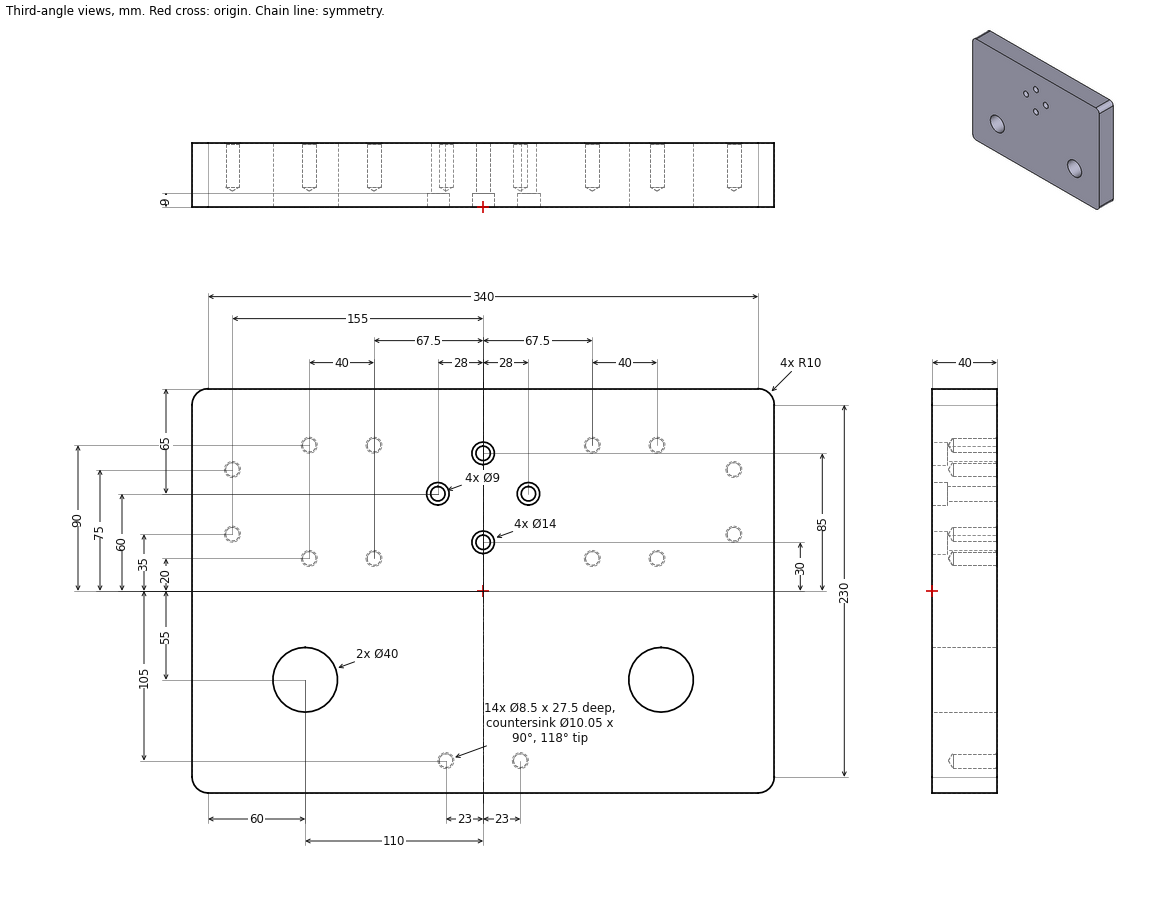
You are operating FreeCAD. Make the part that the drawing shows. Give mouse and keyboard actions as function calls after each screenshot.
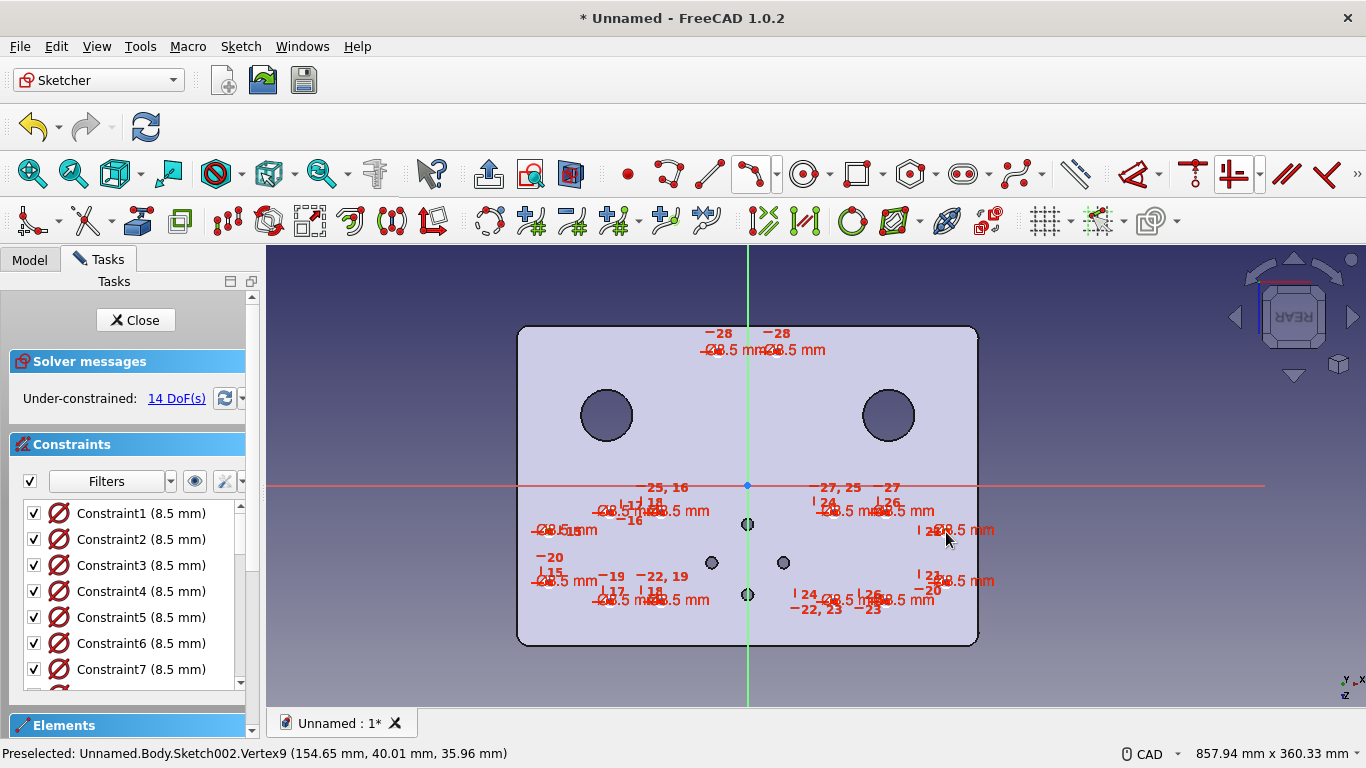
click(748, 650)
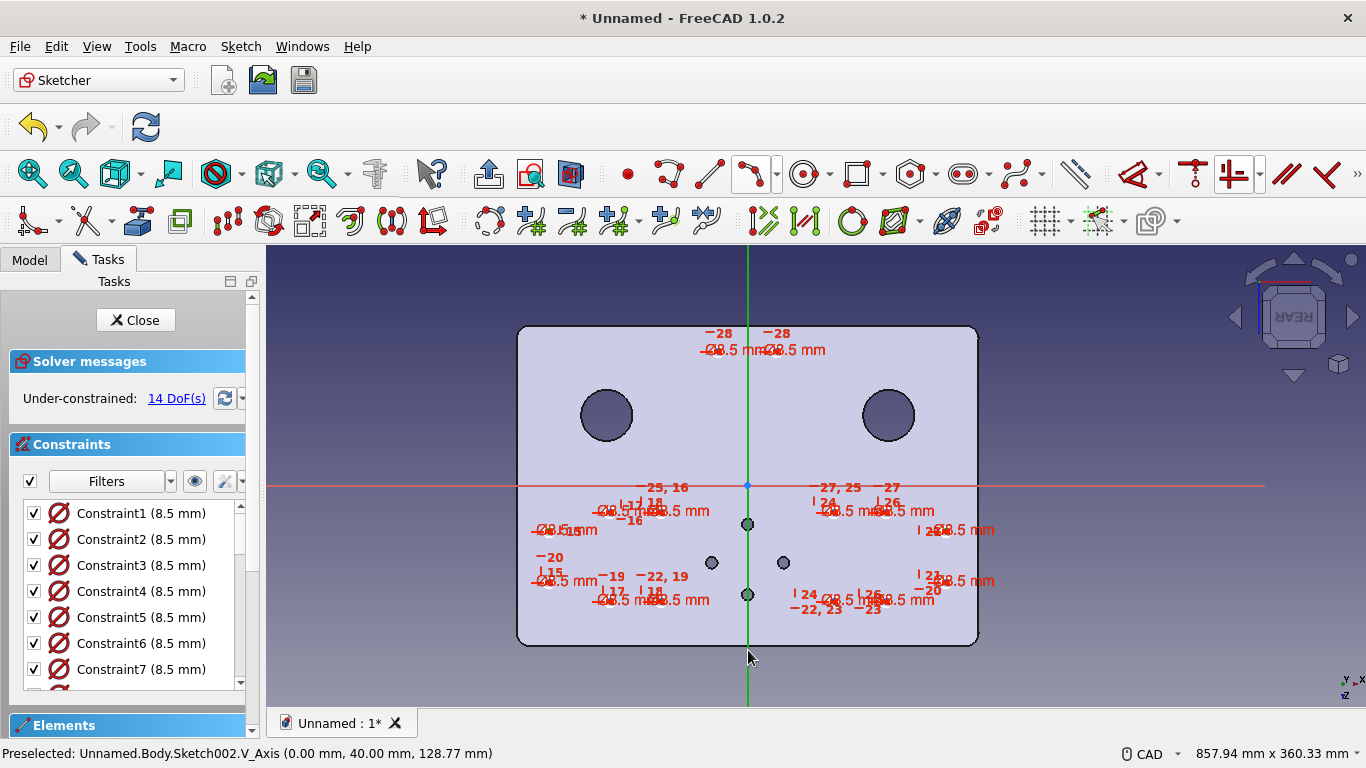
key(s)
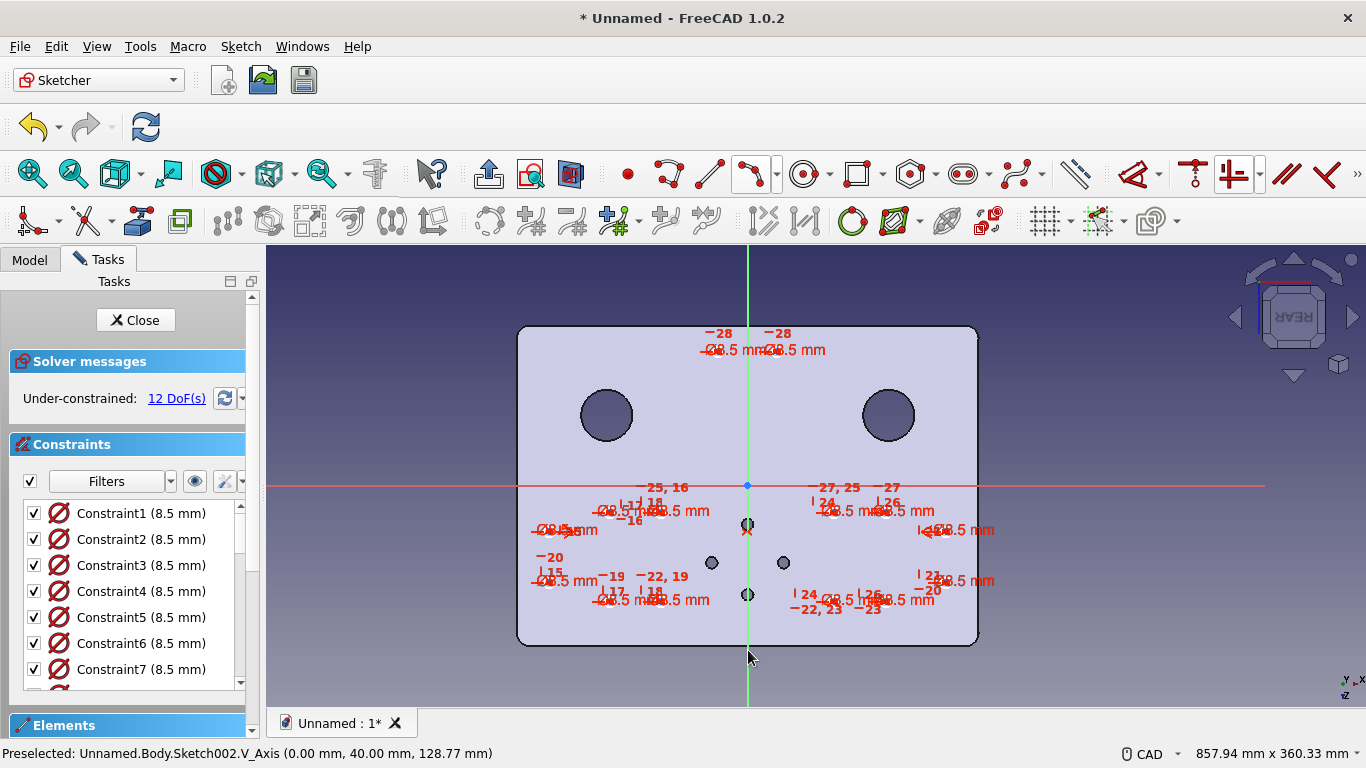
click(1132, 174)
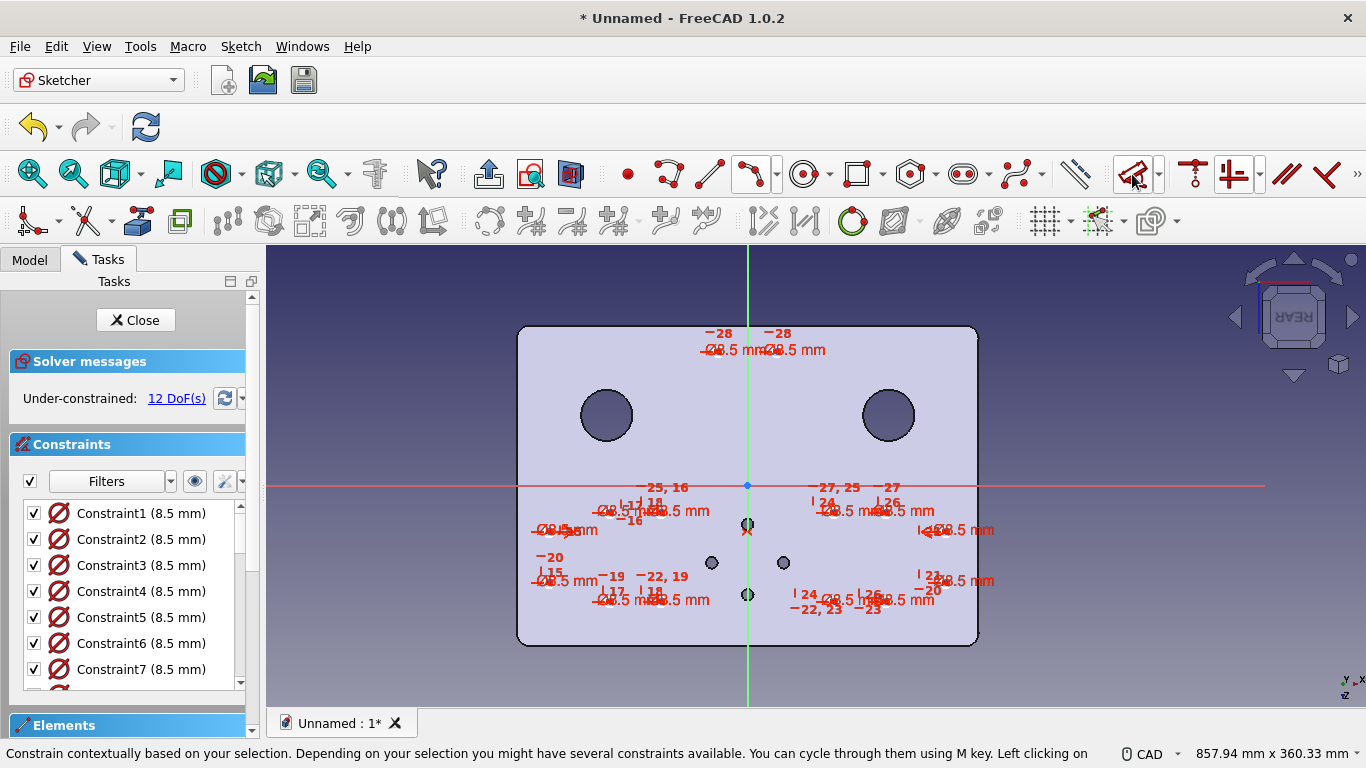
scroll(718, 352, up, 2)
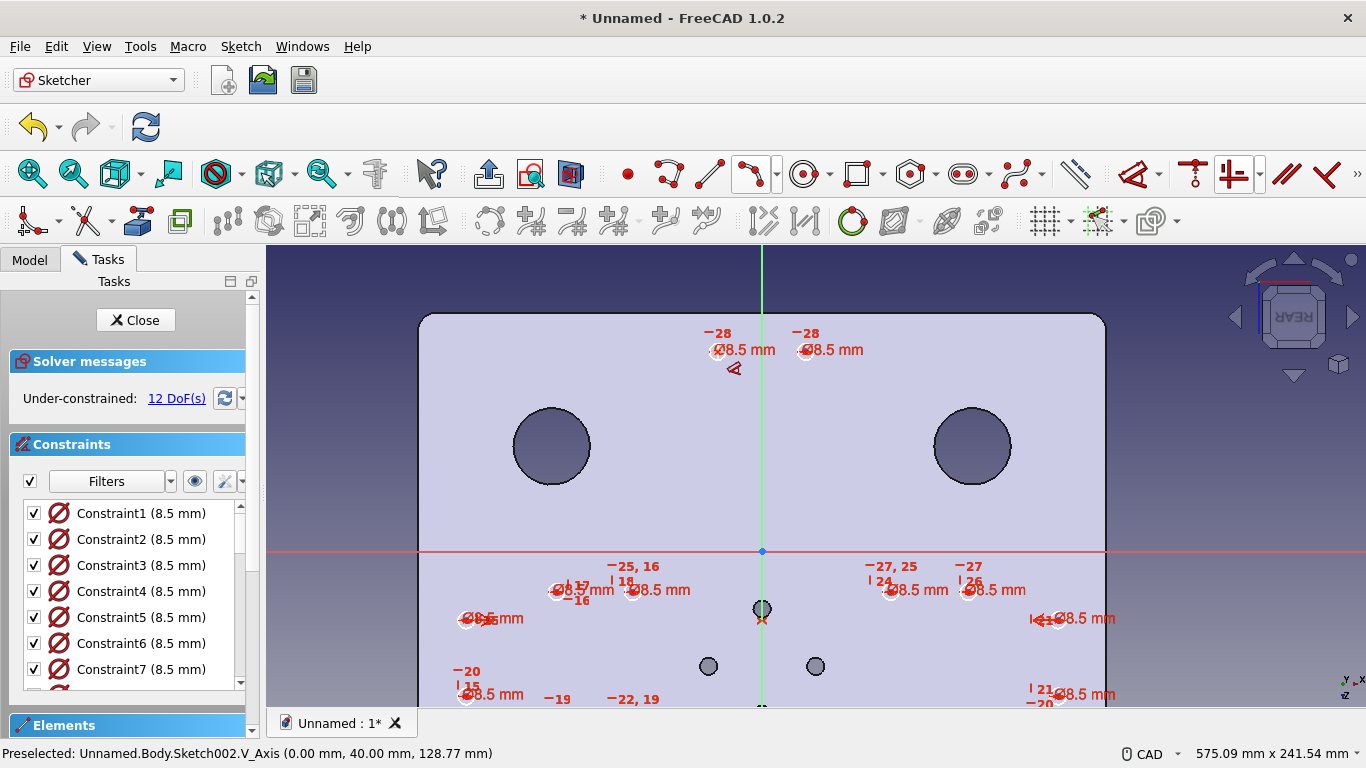
click(718, 352)
click(740, 318)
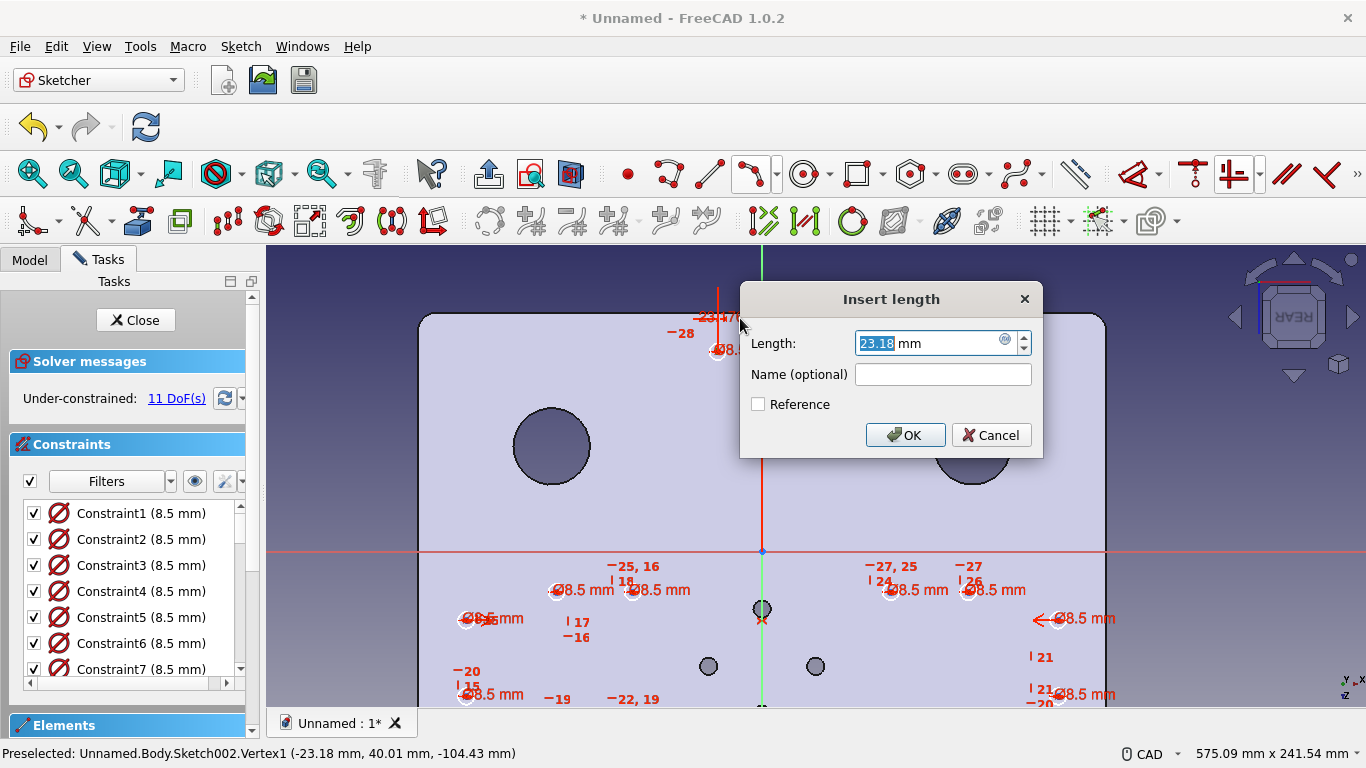
text(23)
key(Return)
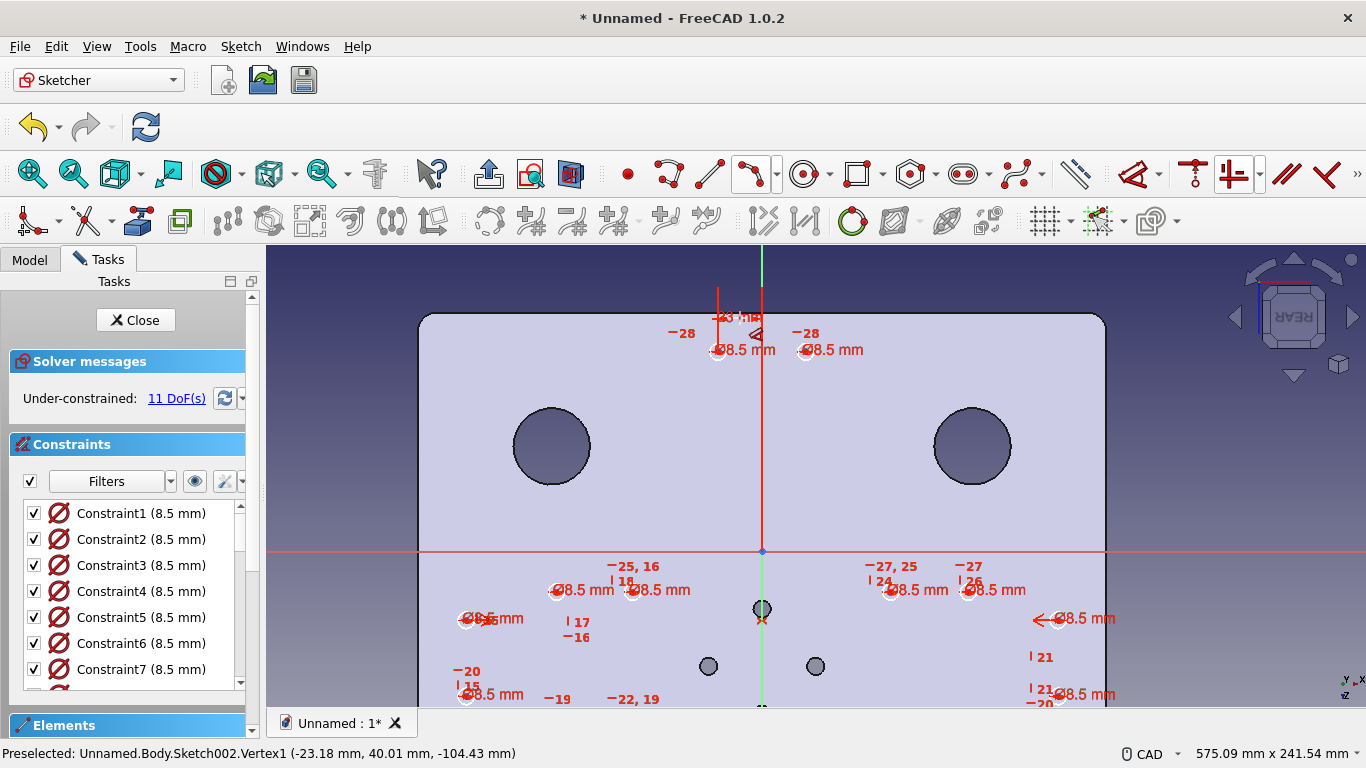
click(466, 620)
click(432, 586)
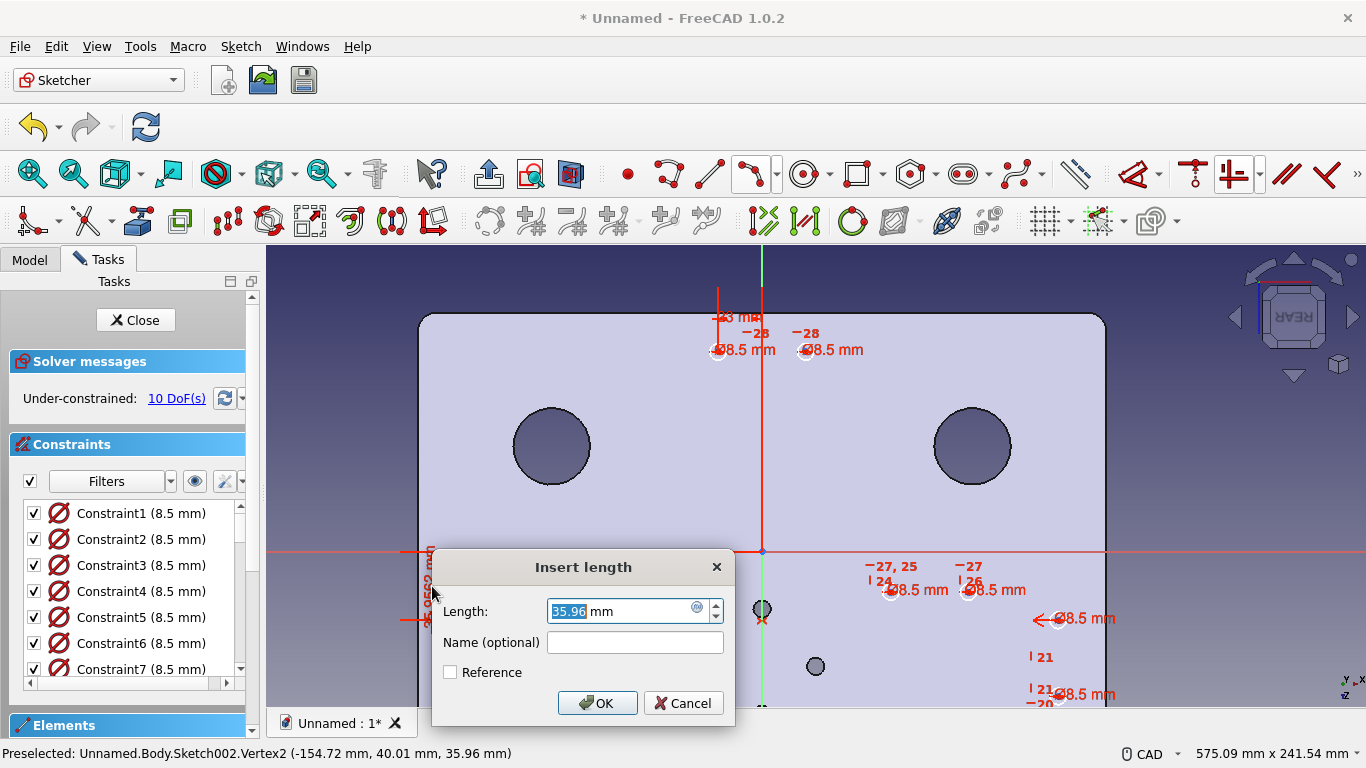
text(35)
key(Return)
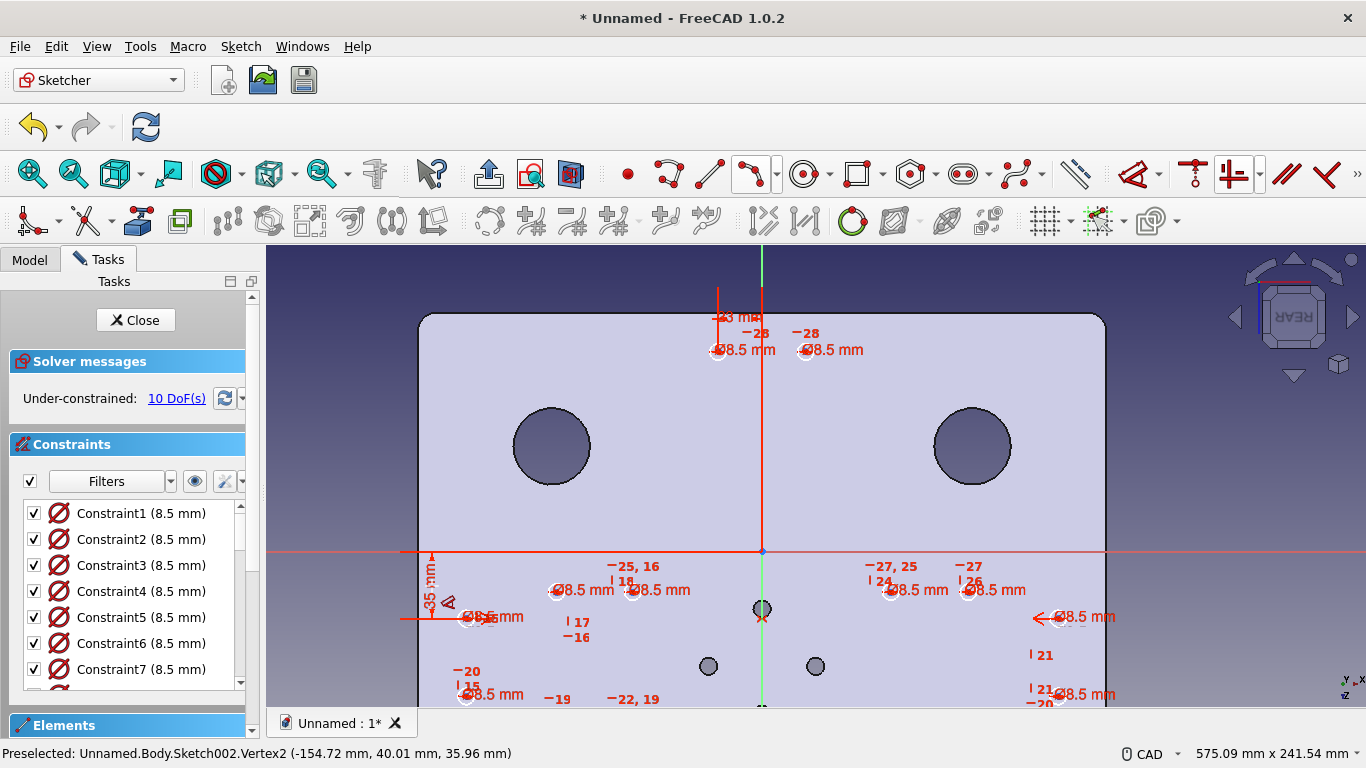
scroll(718, 351, down, 2)